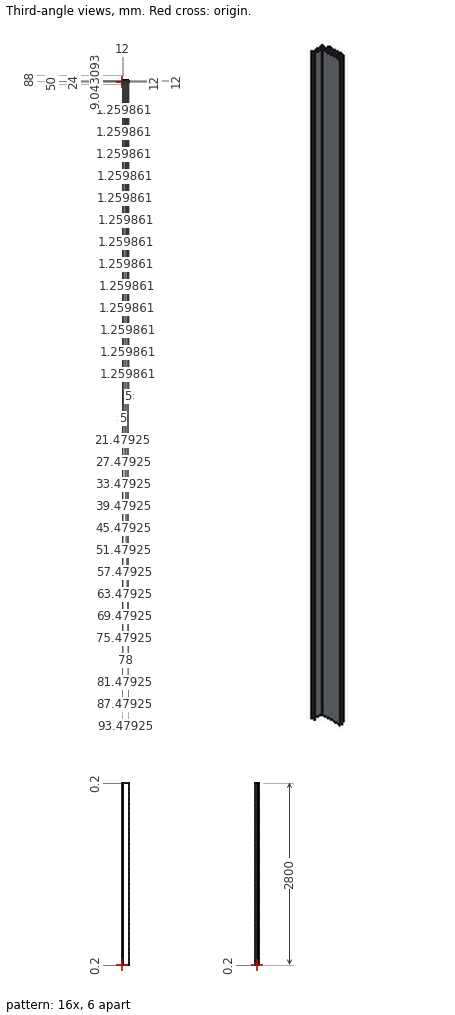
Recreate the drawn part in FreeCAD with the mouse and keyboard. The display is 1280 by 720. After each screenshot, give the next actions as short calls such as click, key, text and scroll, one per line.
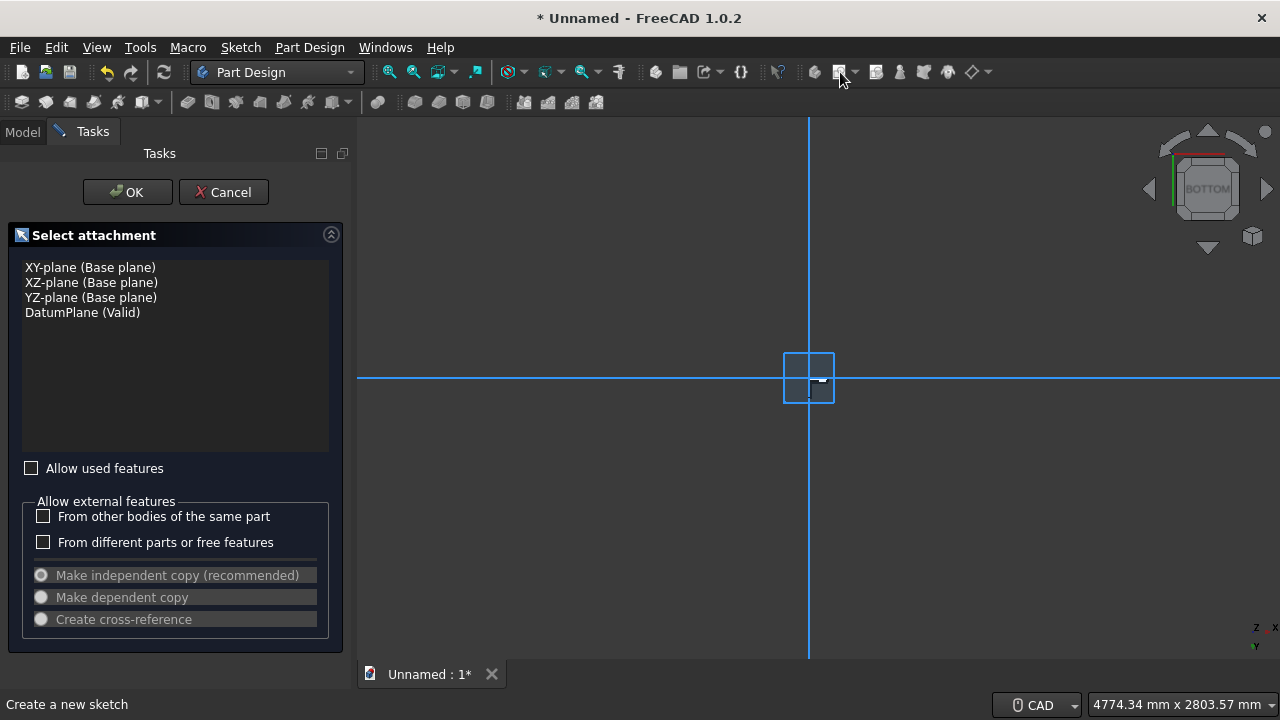
click(82, 268)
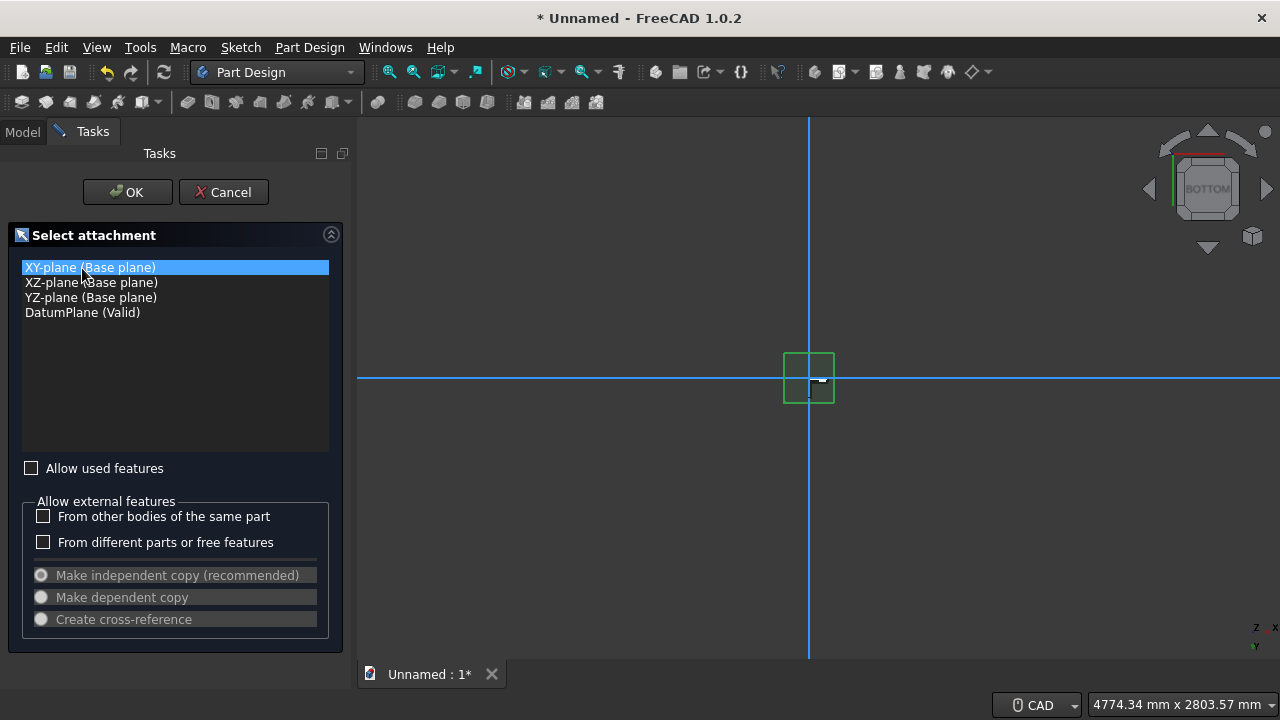
click(128, 192)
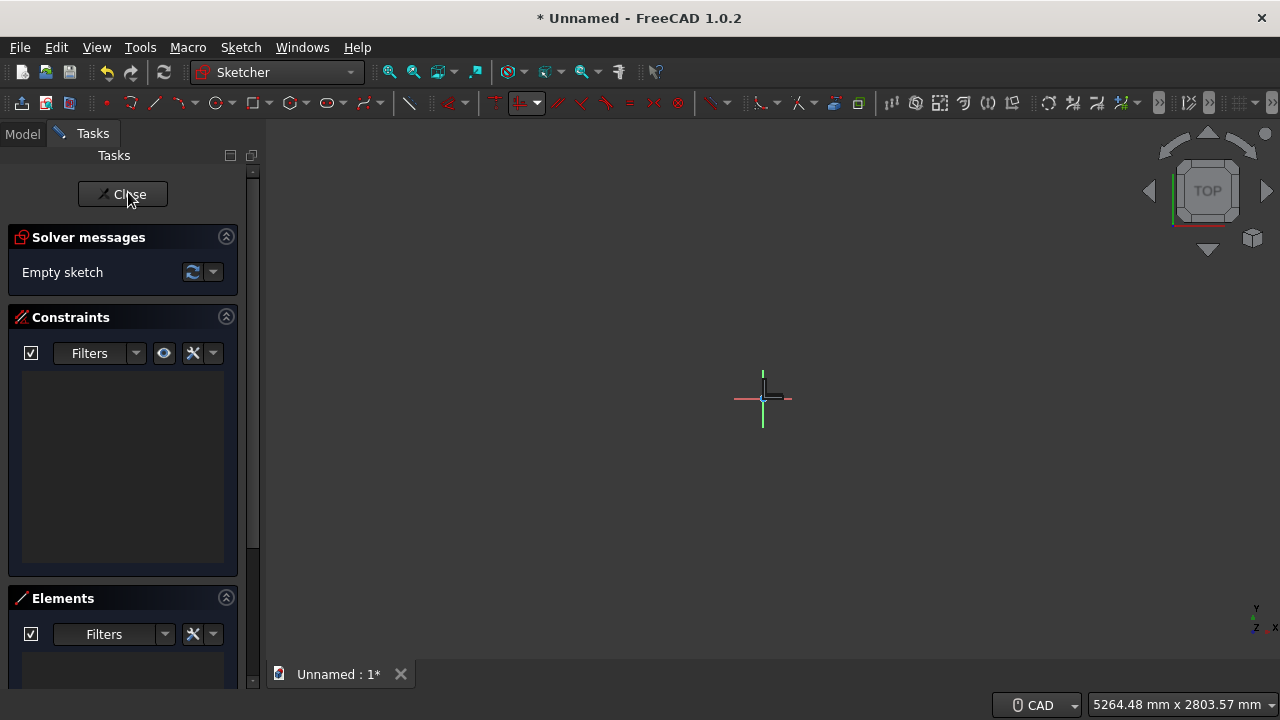
click(70, 104)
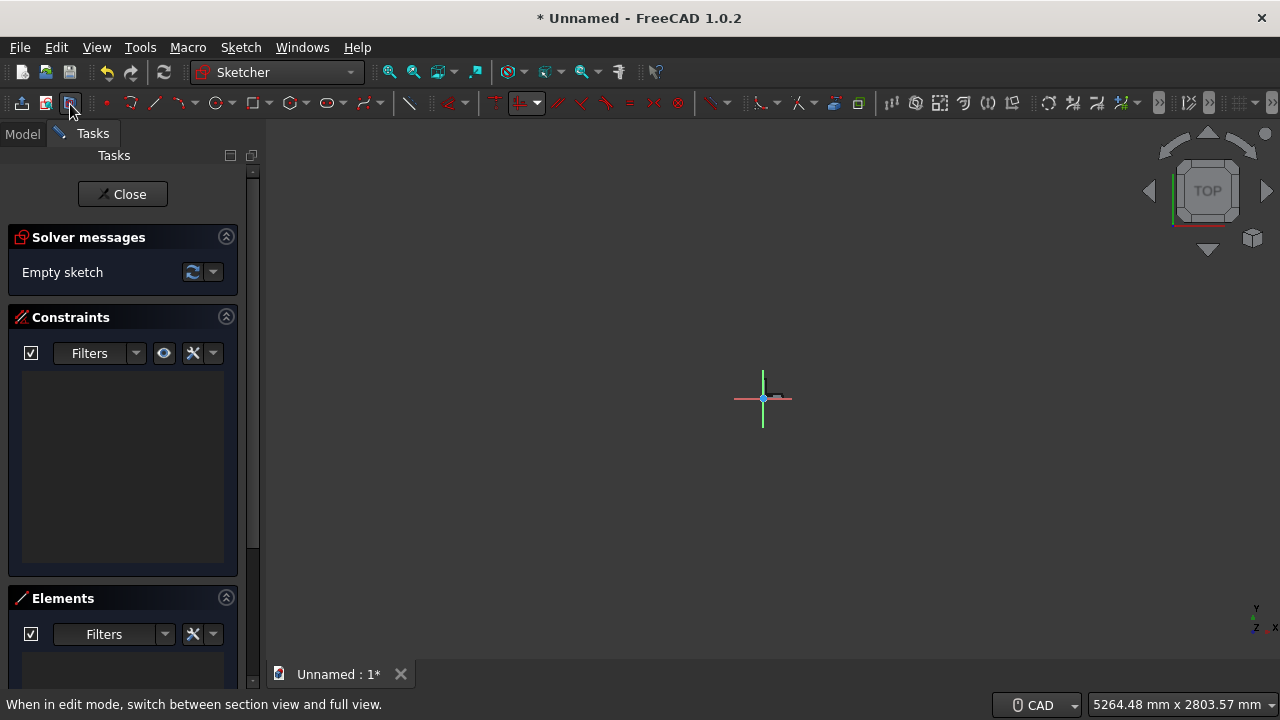
scroll(777, 395, up, 15)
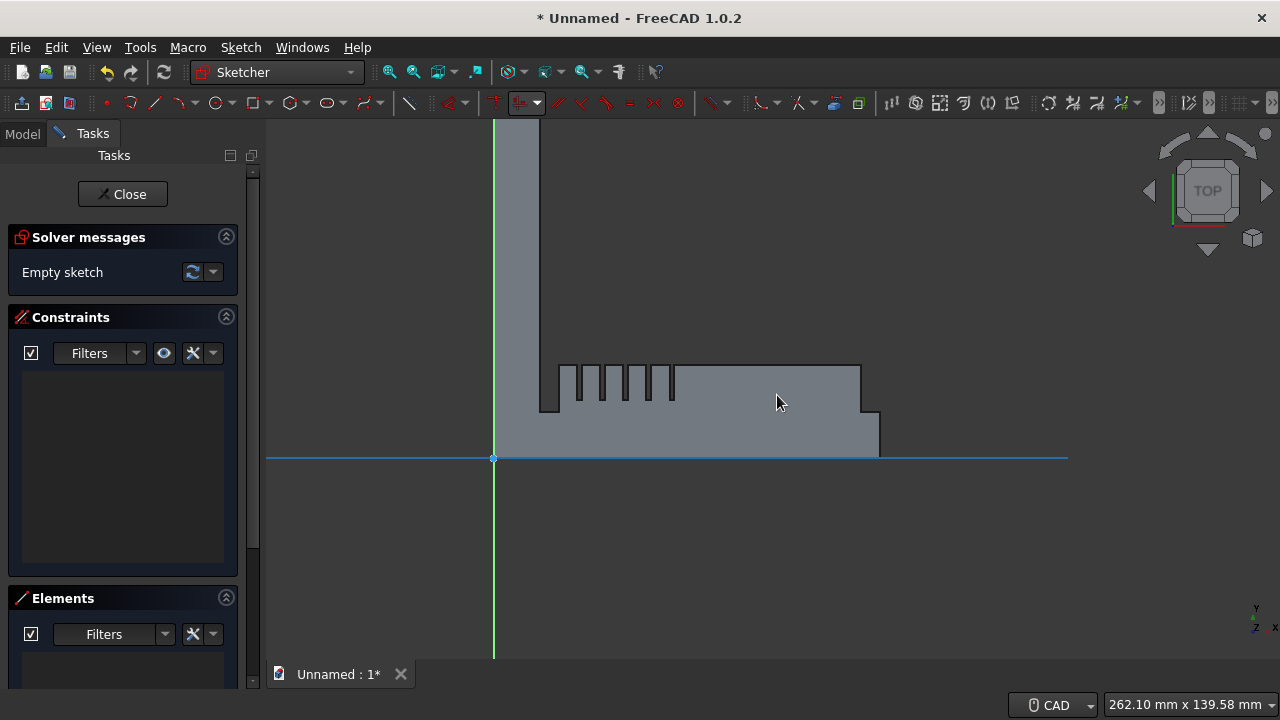
scroll(694, 382, up, 11)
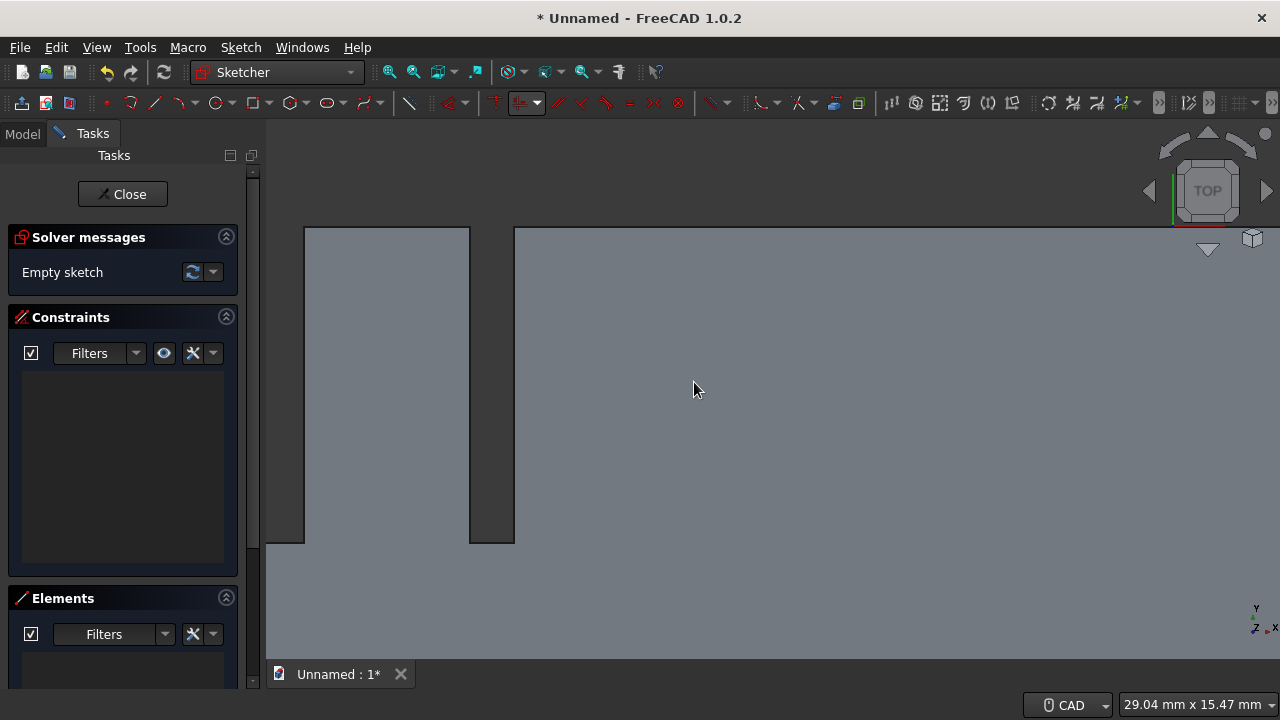
click(254, 104)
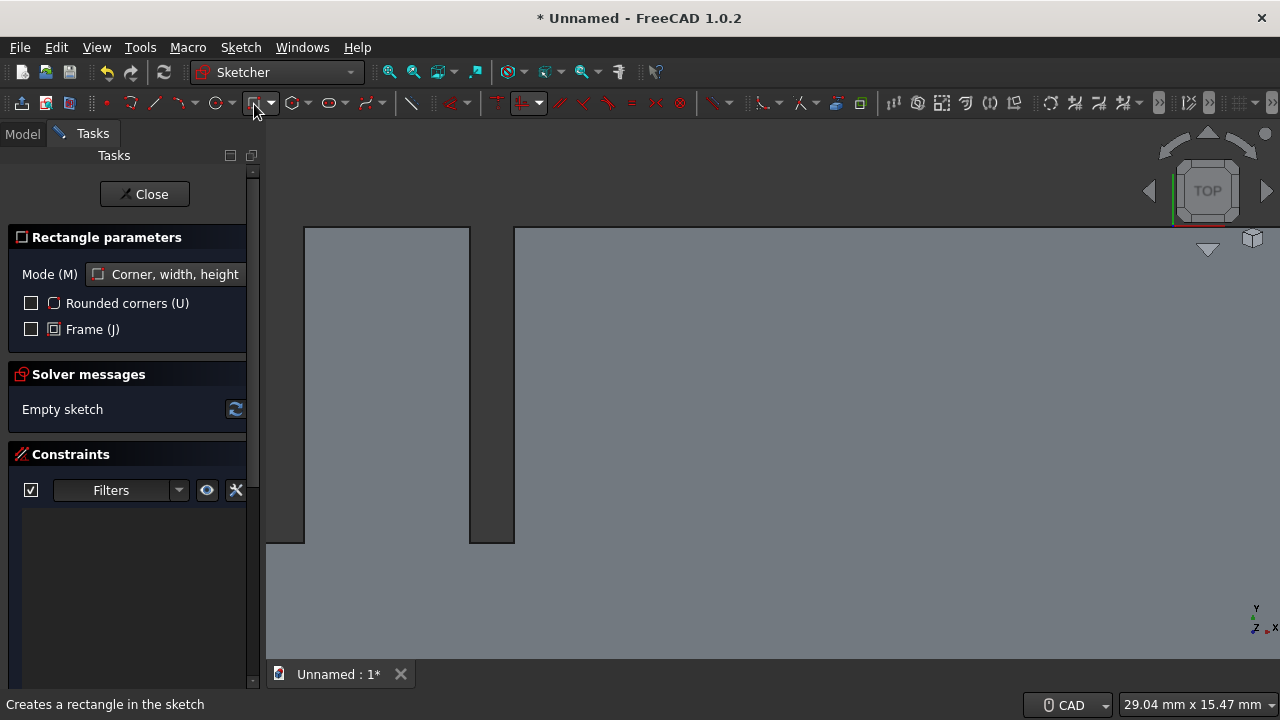
click(679, 227)
move(723, 543)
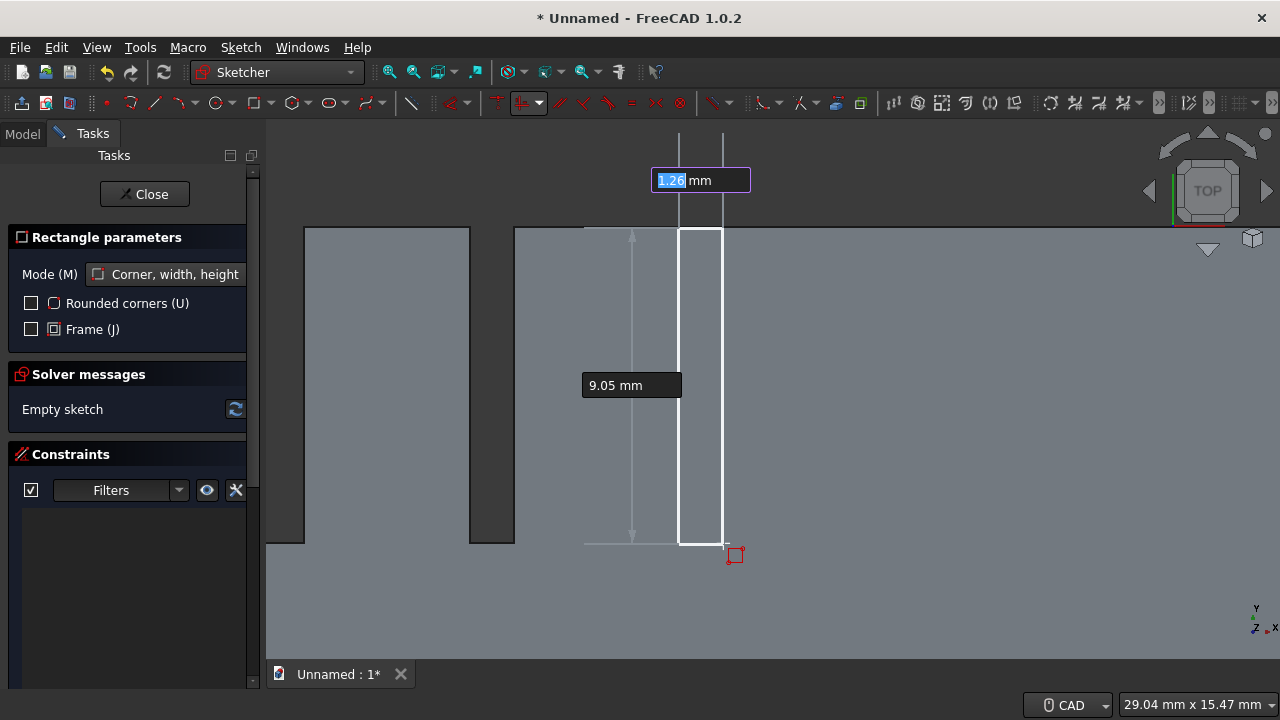
text(1.259861)
key(Tab)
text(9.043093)
key(Return)
key(Escape)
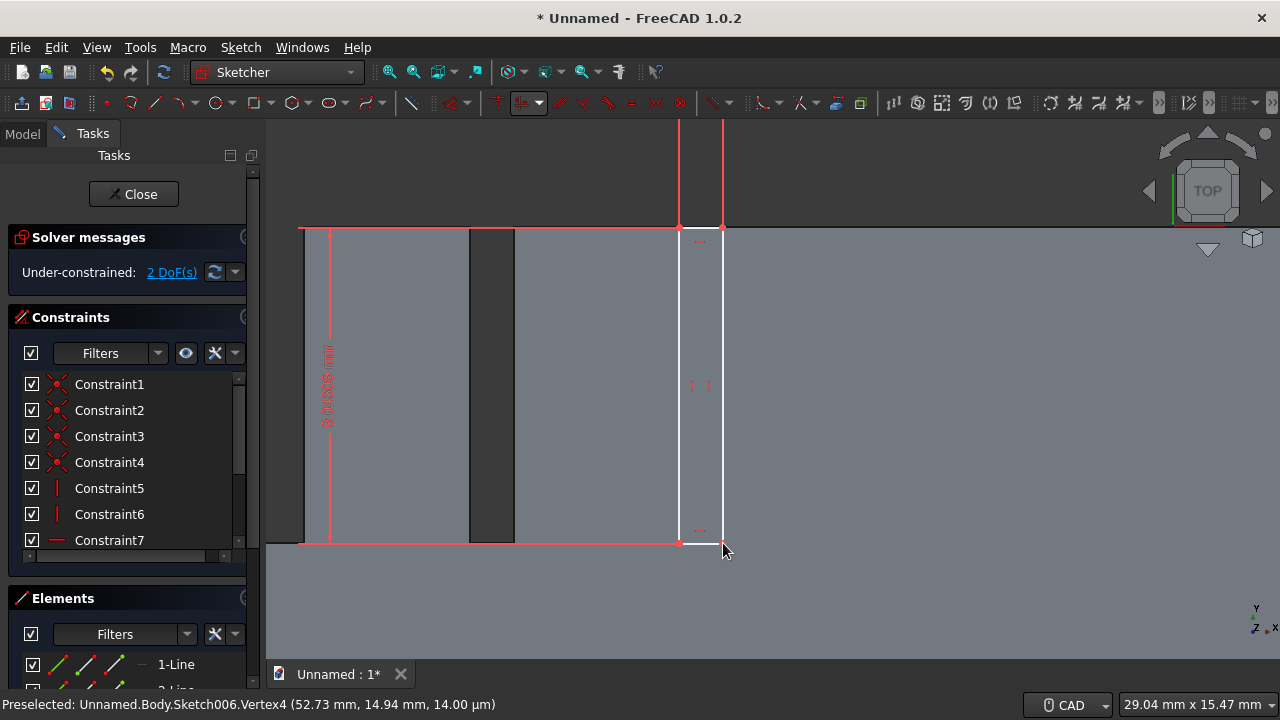
click(450, 104)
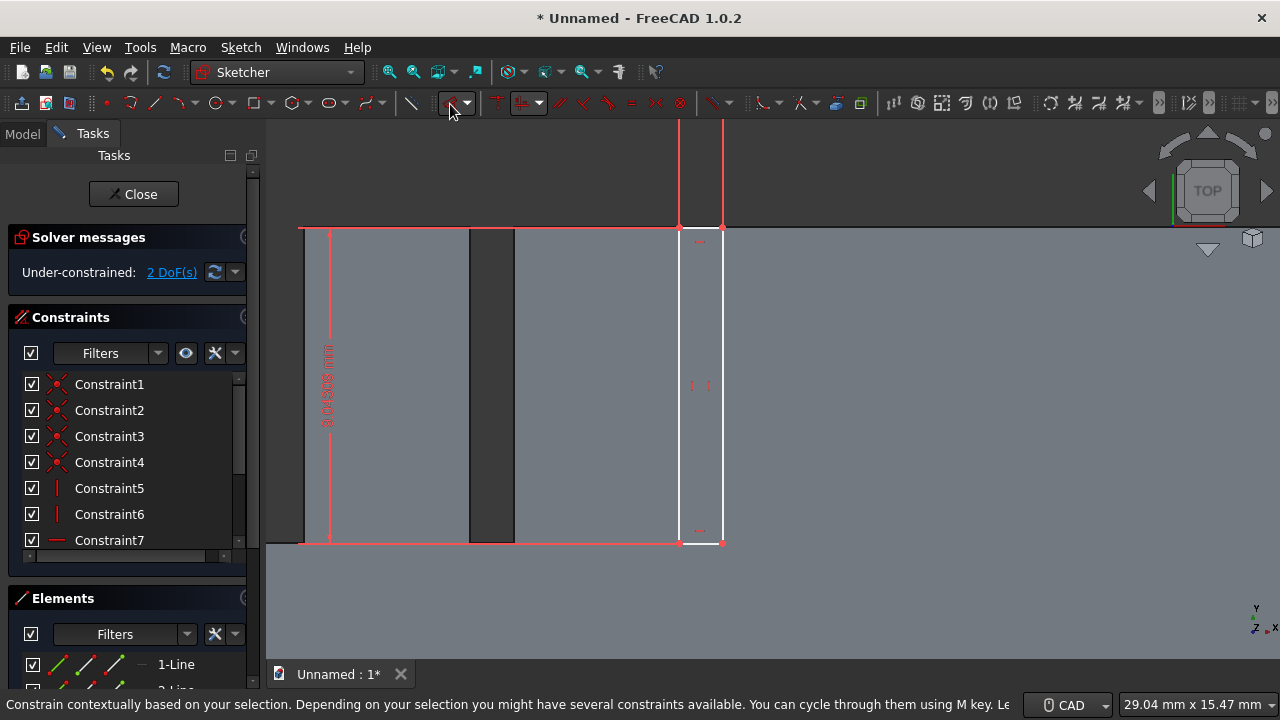
click(679, 228)
click(713, 571)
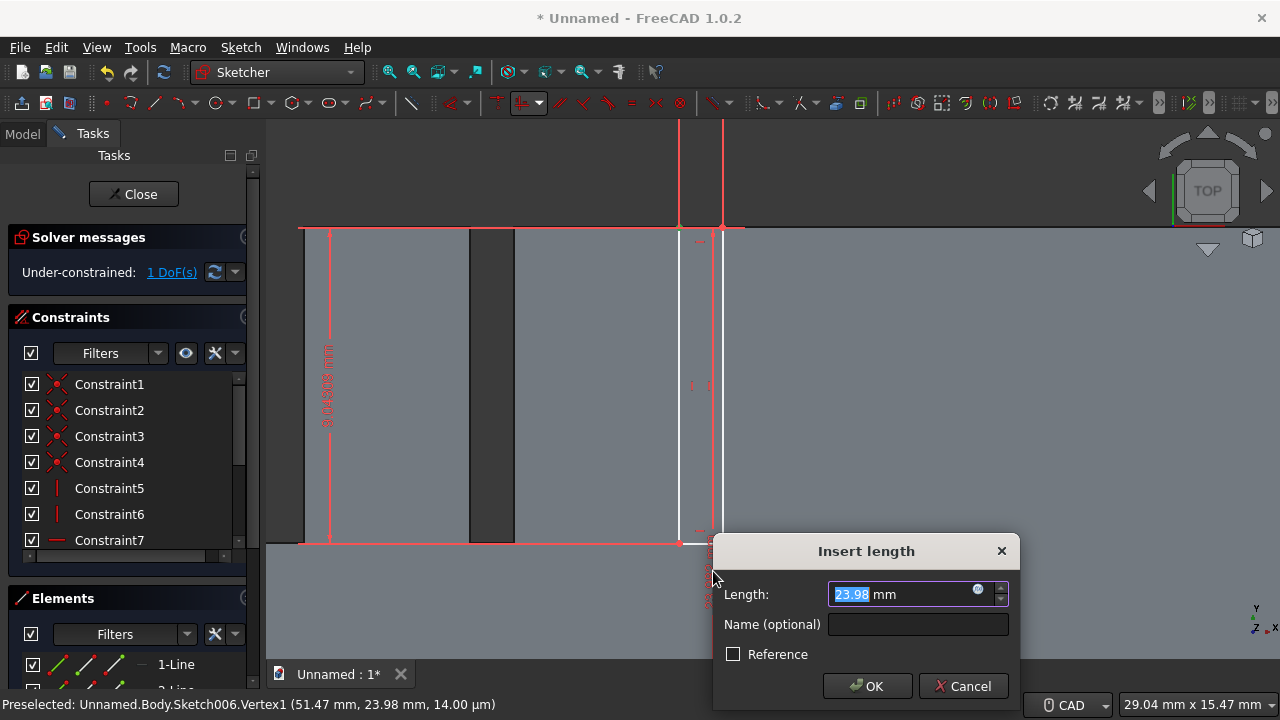
text(24)
key(Return)